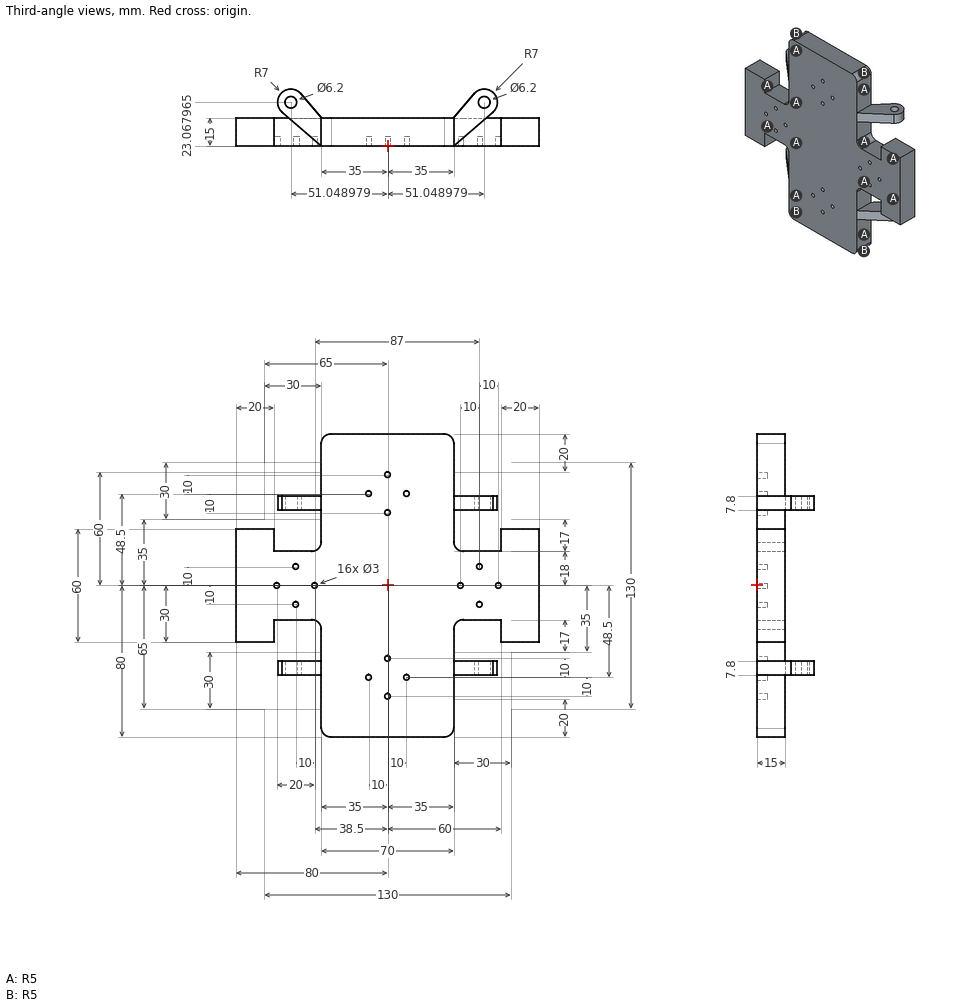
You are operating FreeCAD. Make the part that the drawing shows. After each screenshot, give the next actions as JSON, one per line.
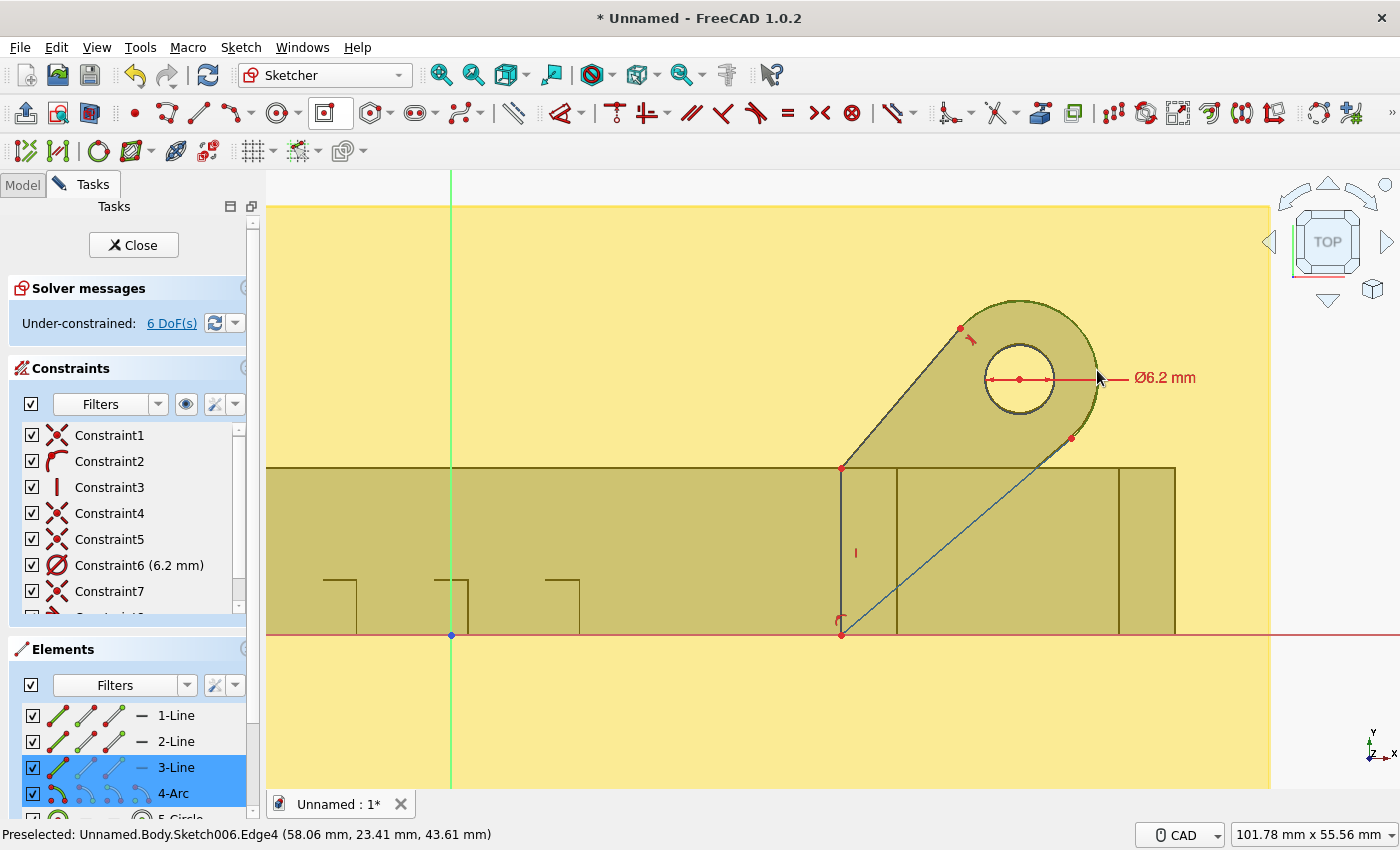
{"action": "key", "text": "t"}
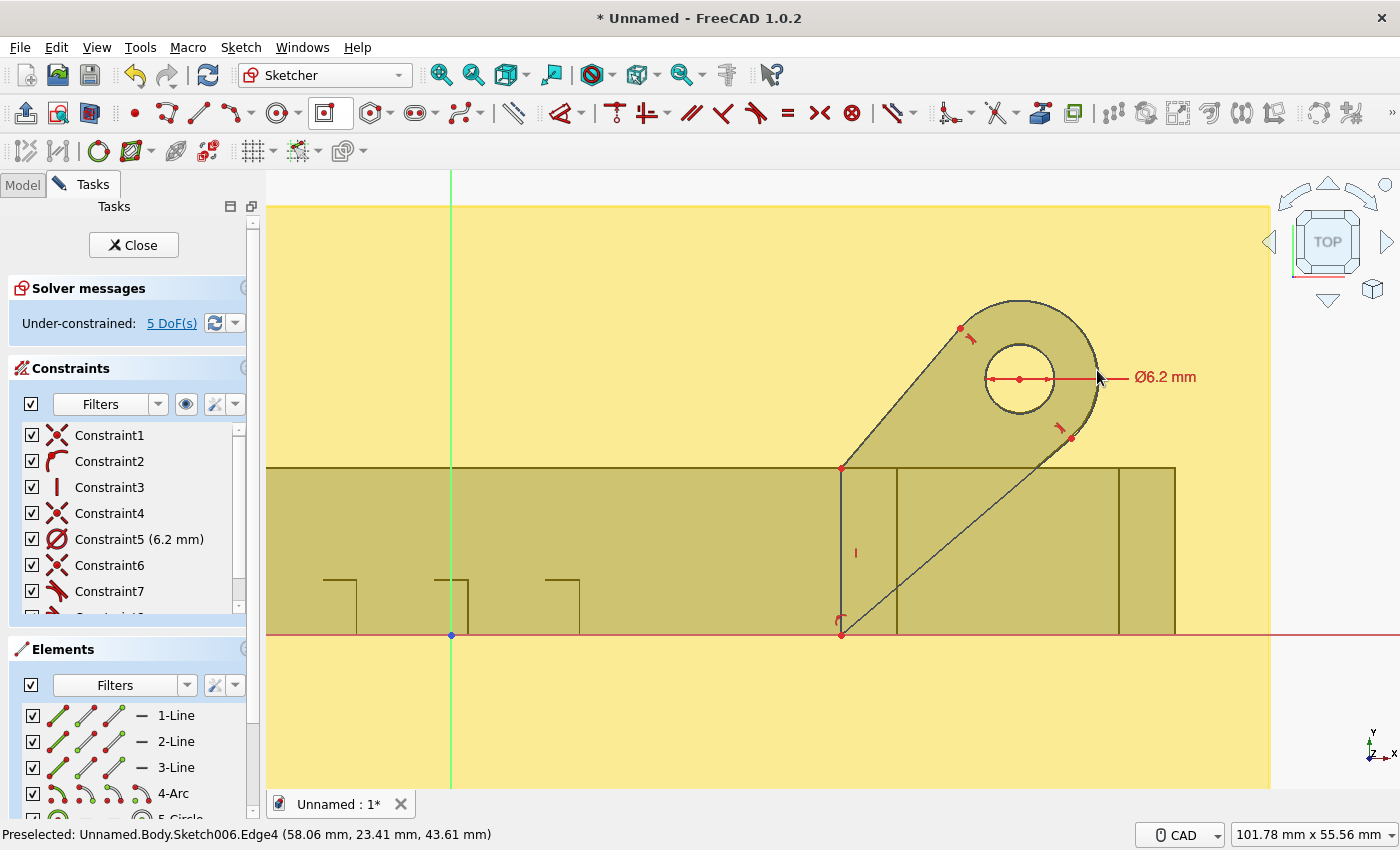
{"action": "key", "text": "d"}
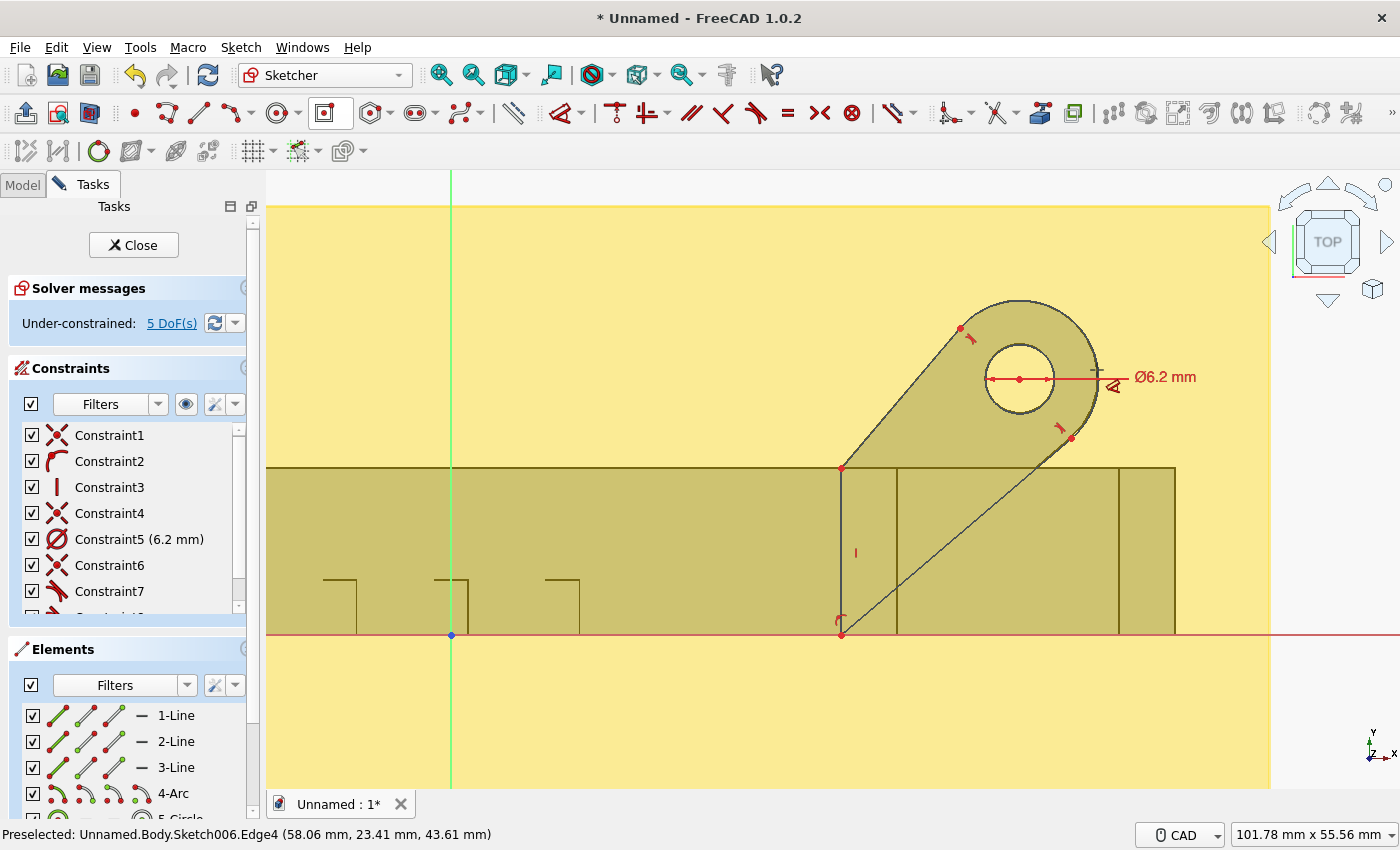
{"action": "left_click", "coordinate": [1098, 369]}
{"action": "left_click", "coordinate": [1130, 365]}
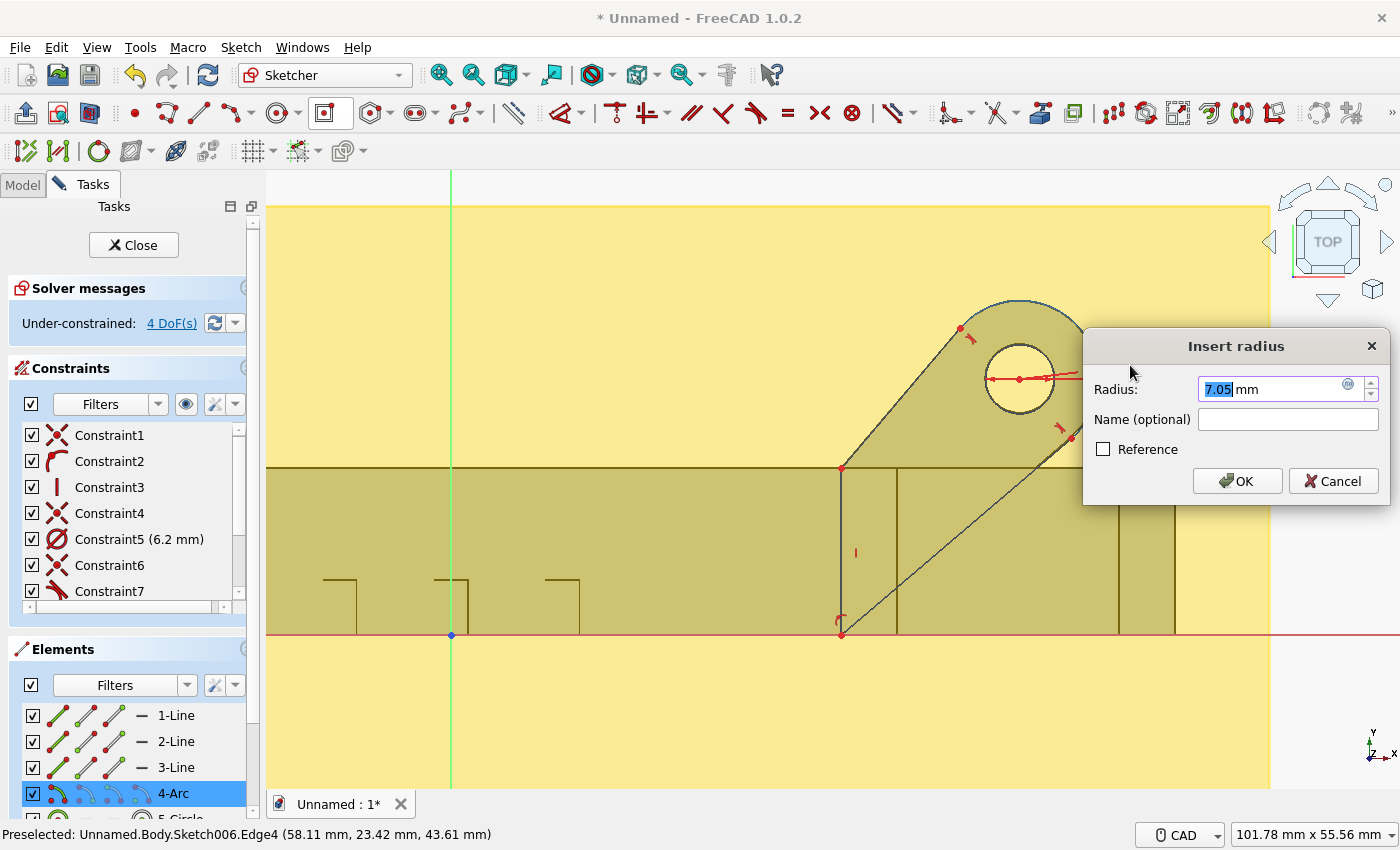
{"action": "type", "text": "7"}
{"action": "key", "text": "Return"}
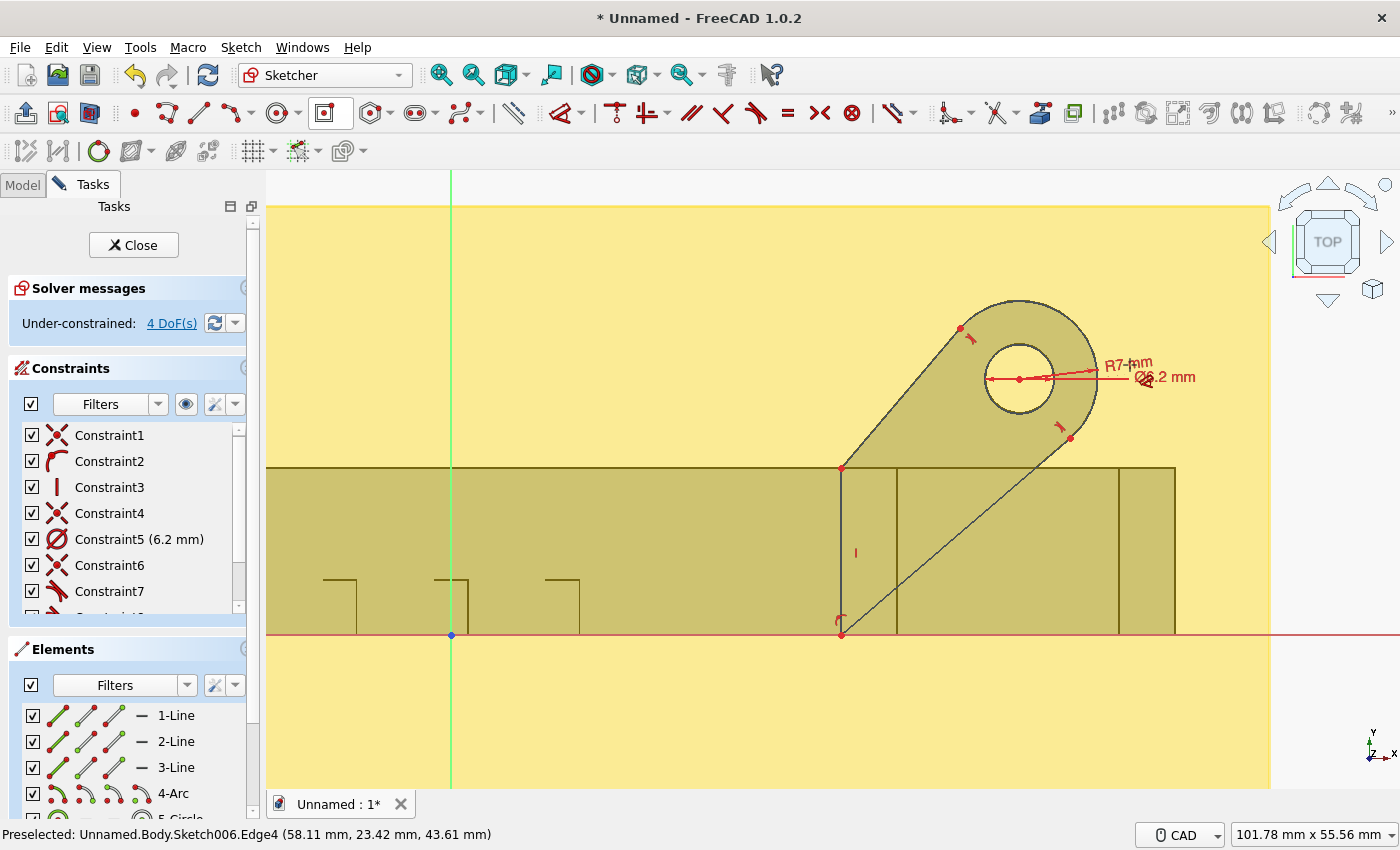
{"action": "left_click", "coordinate": [841, 519]}
{"action": "left_click", "coordinate": [875, 552]}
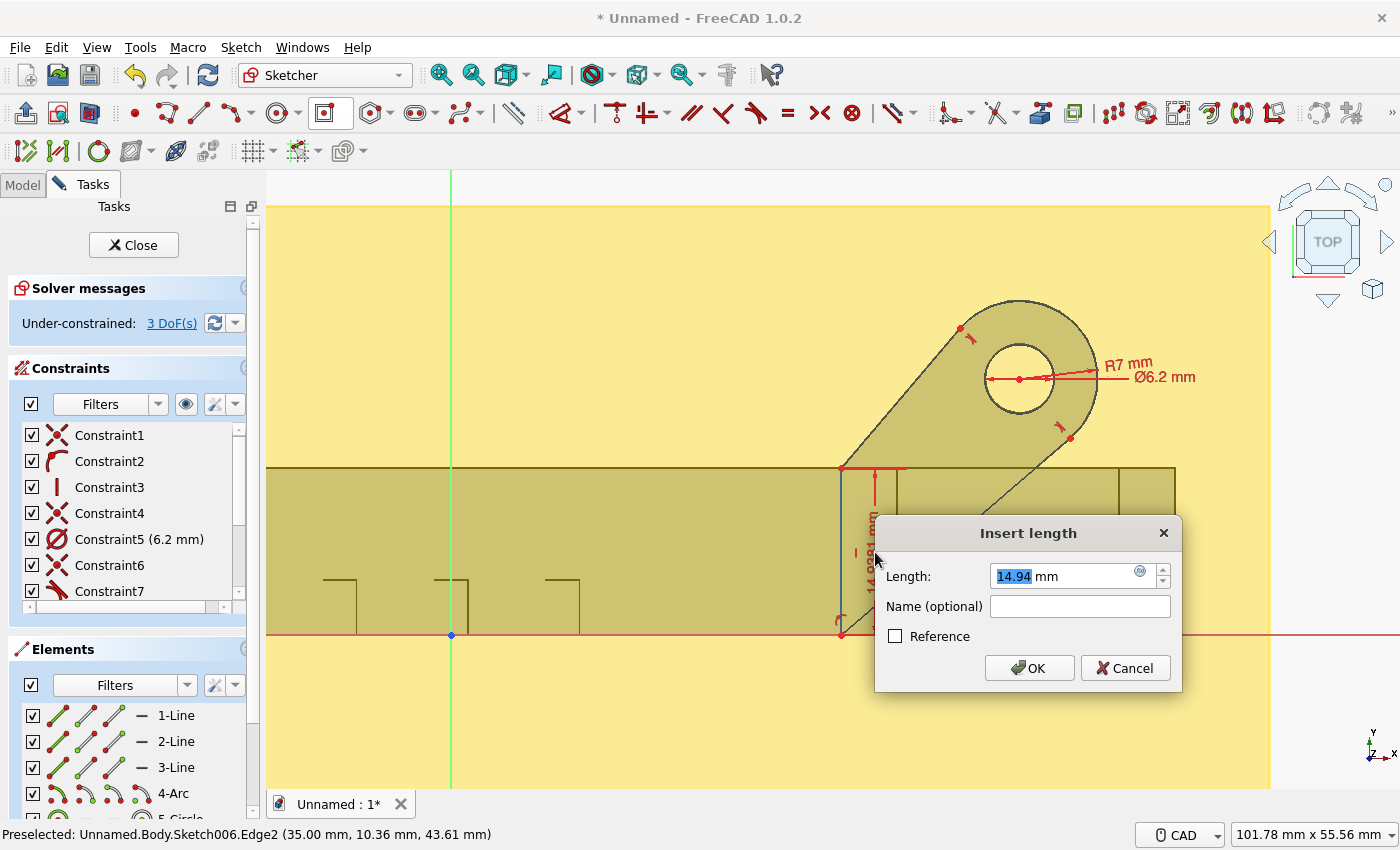
{"action": "type", "text": "15"}
{"action": "key", "text": "Return"}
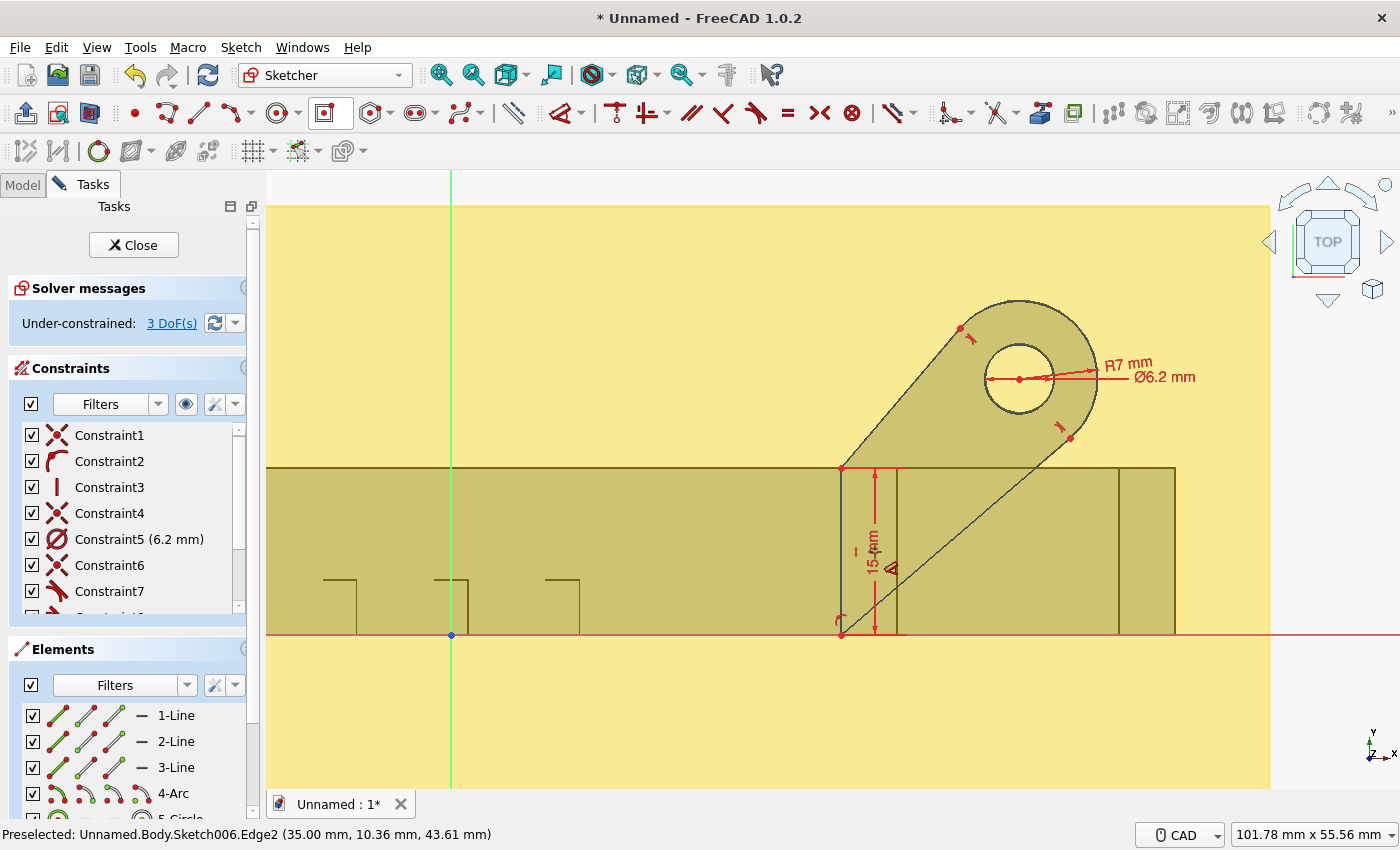
{"action": "left_click", "coordinate": [841, 468]}
{"action": "left_click", "coordinate": [646, 669]}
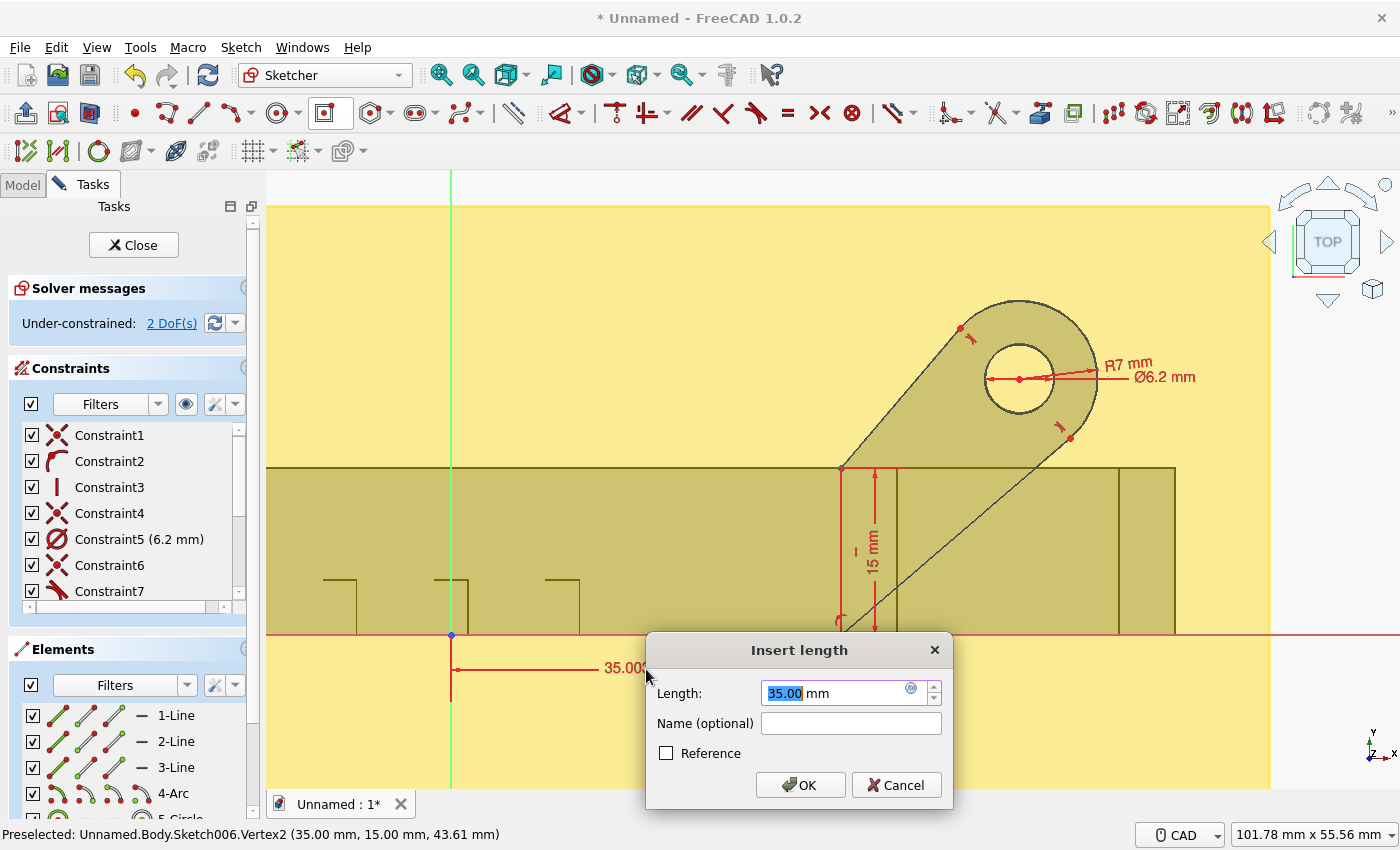
{"action": "type", "text": "35"}
{"action": "key", "text": "Return"}